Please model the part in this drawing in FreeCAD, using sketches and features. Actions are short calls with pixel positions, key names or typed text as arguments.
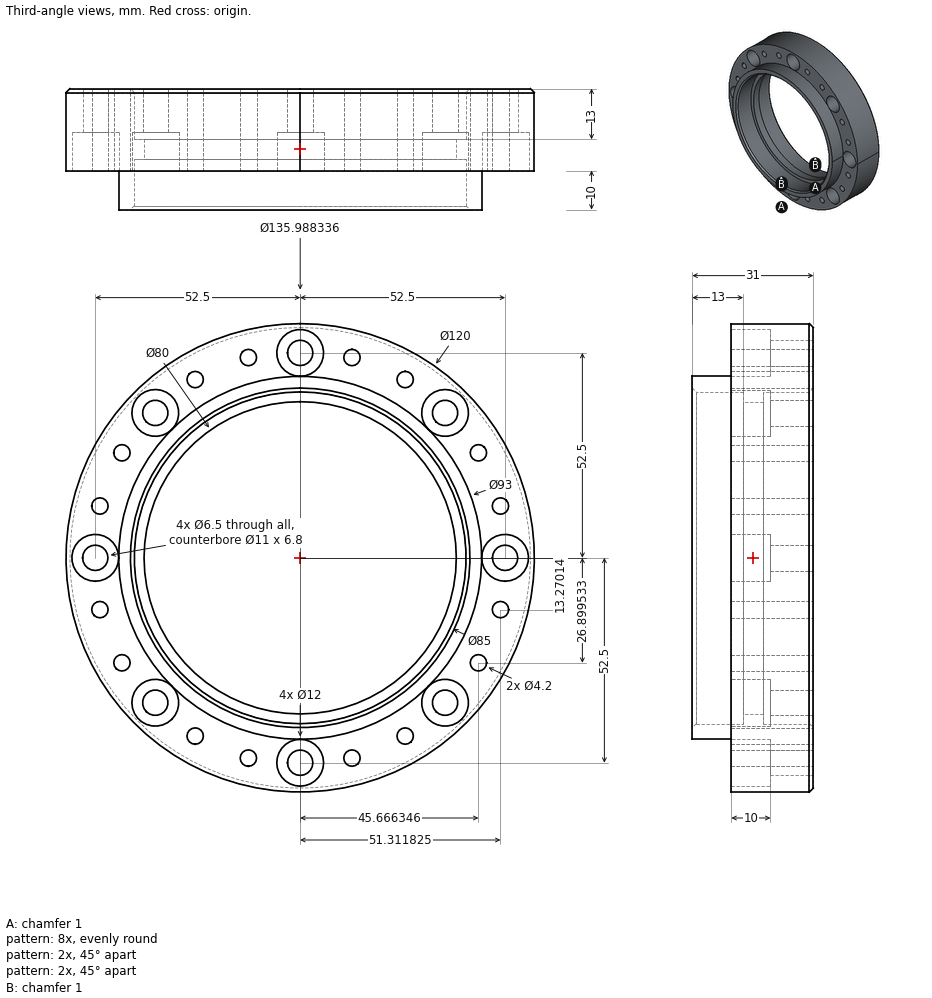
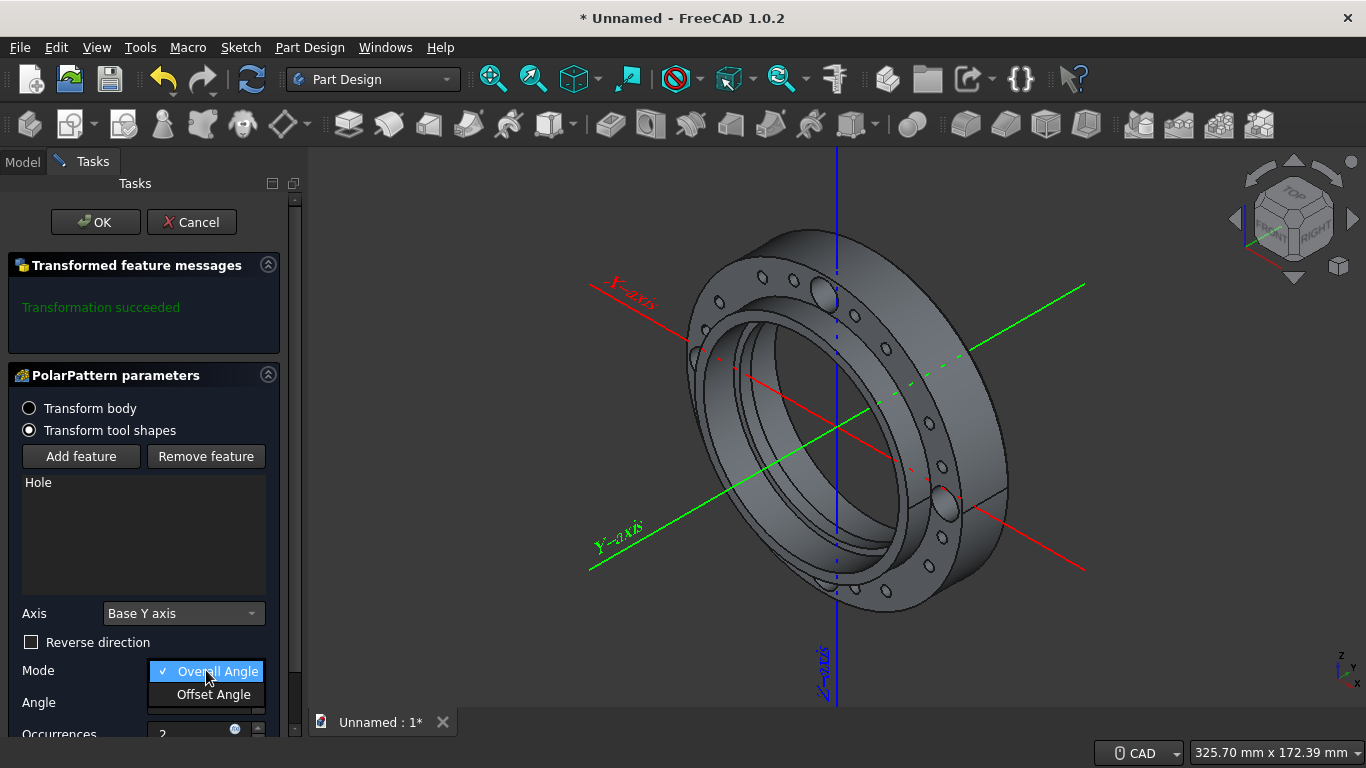
click(206, 694)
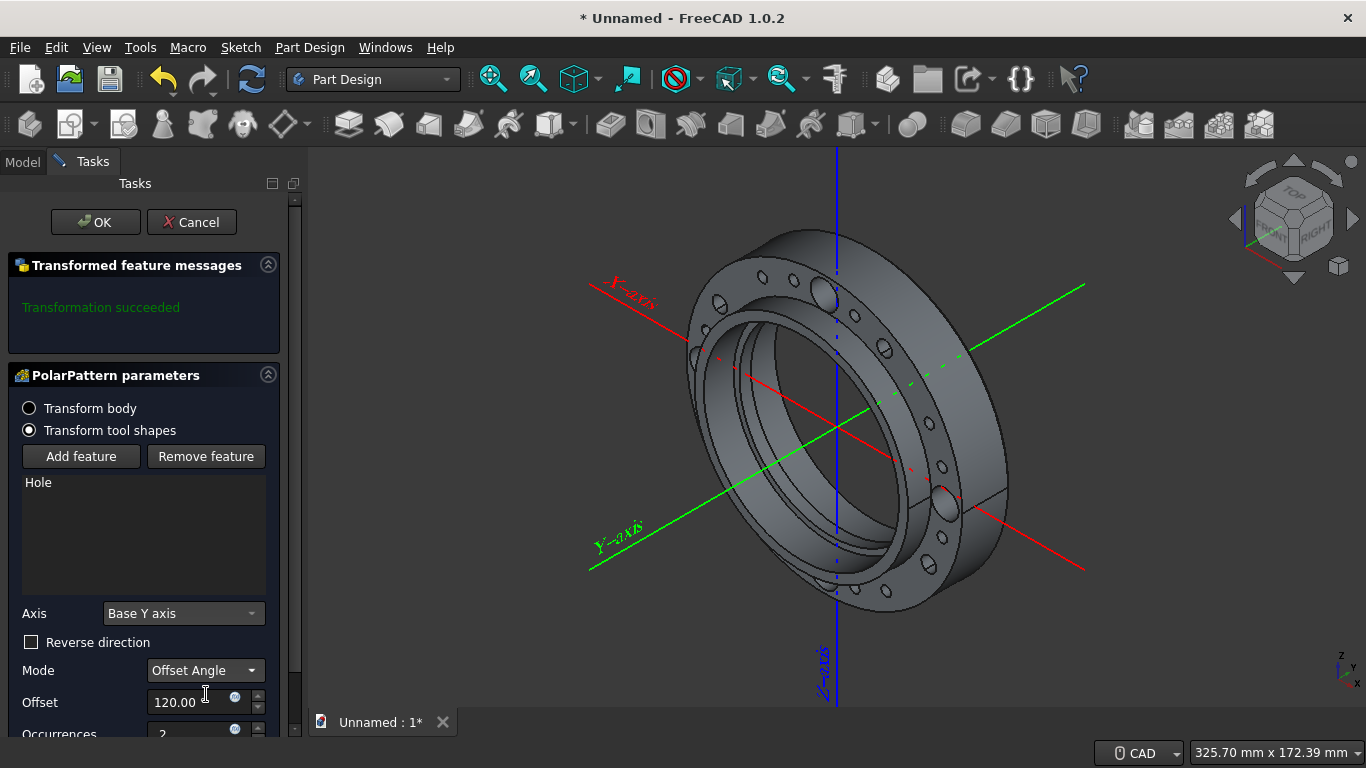
triple_click(198, 702)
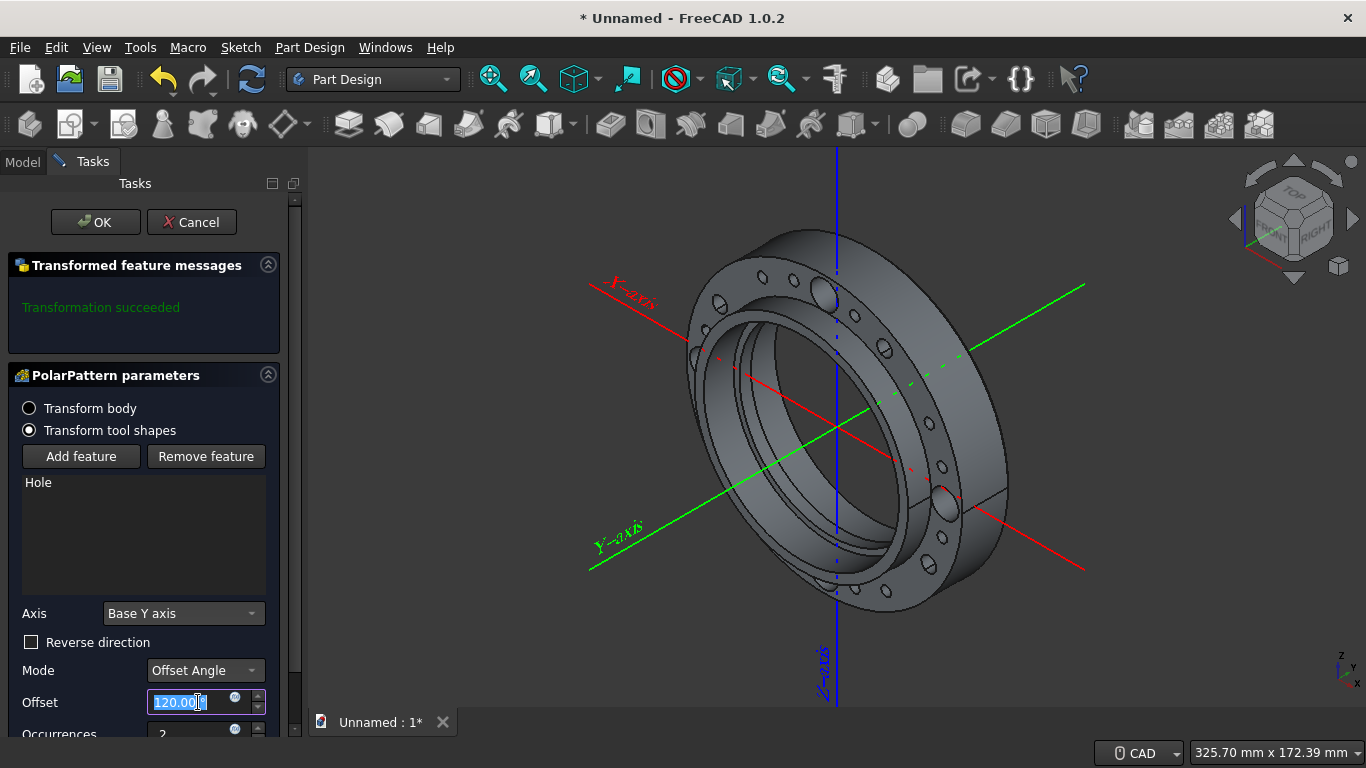
text(45)
key(Tab)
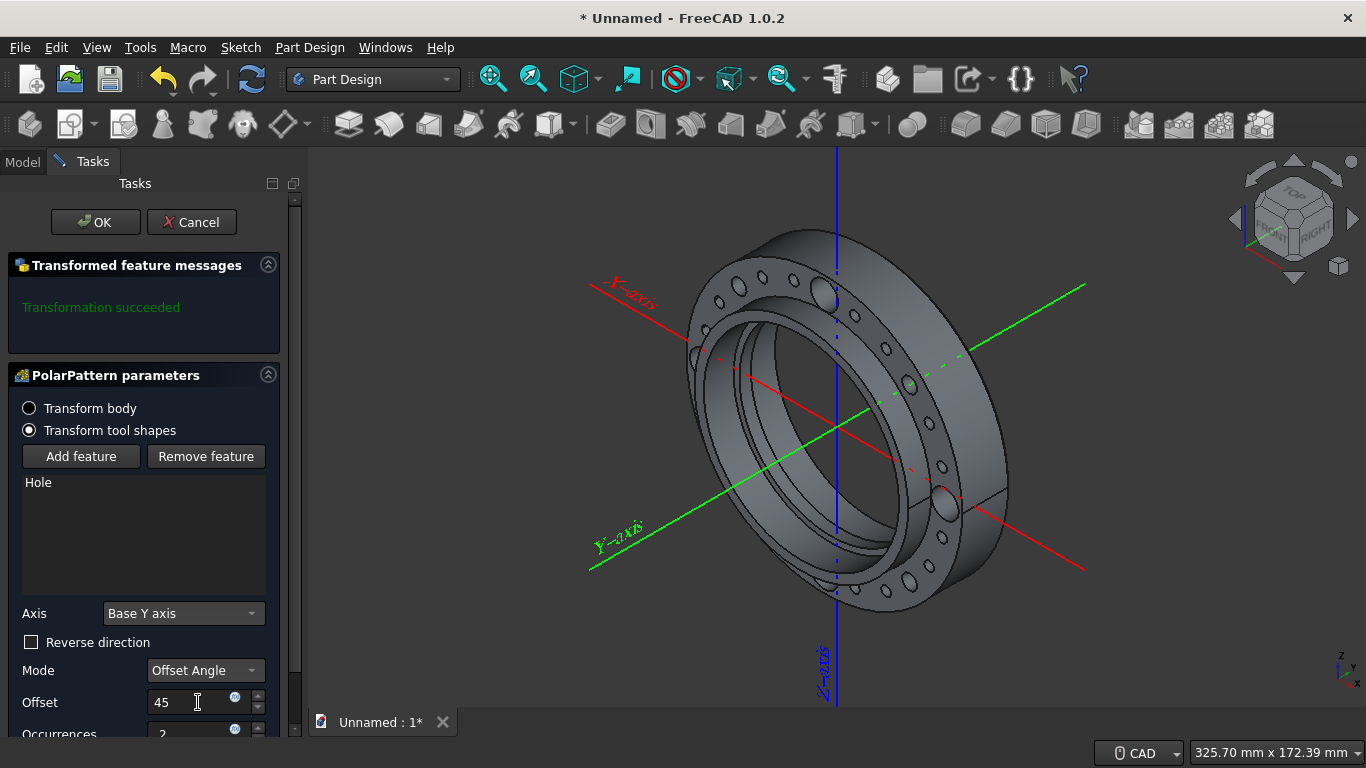
scroll(295, 464, down, 2)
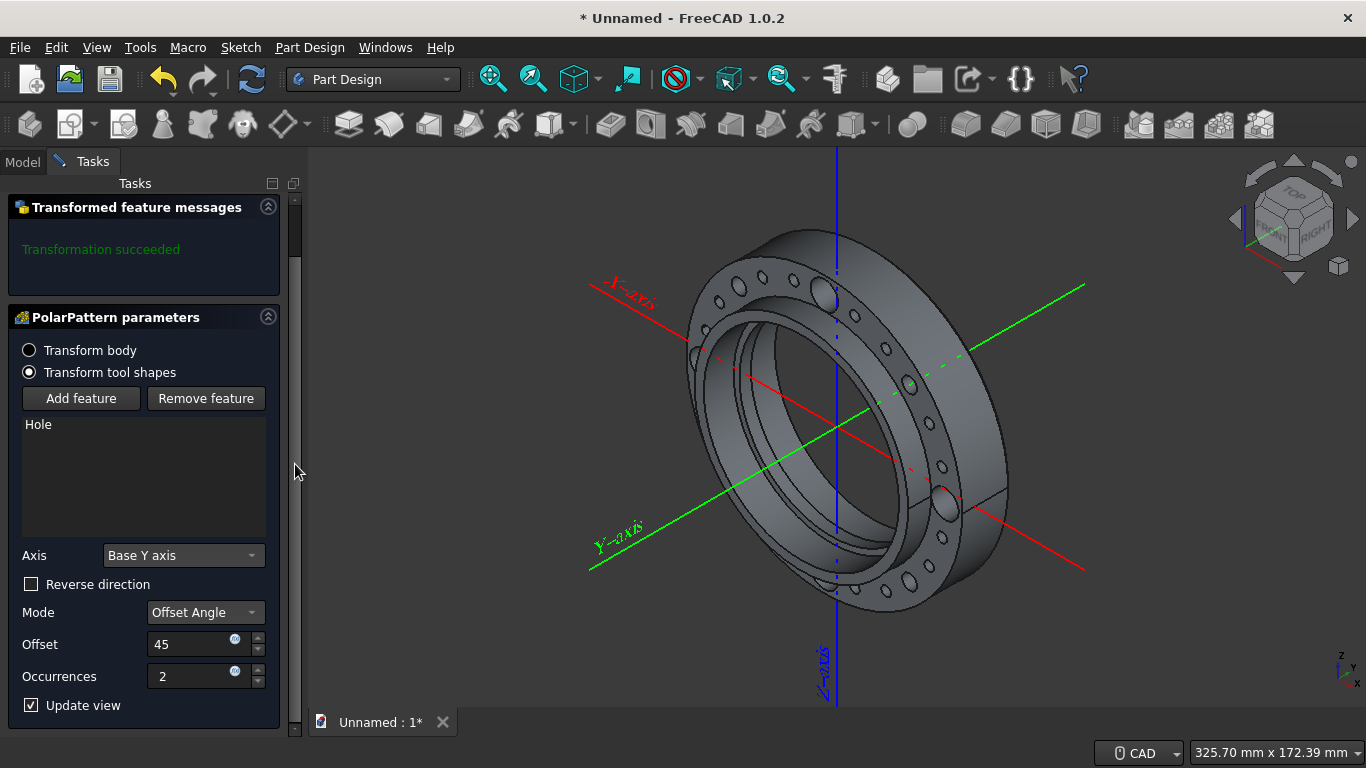
triple_click(198, 676)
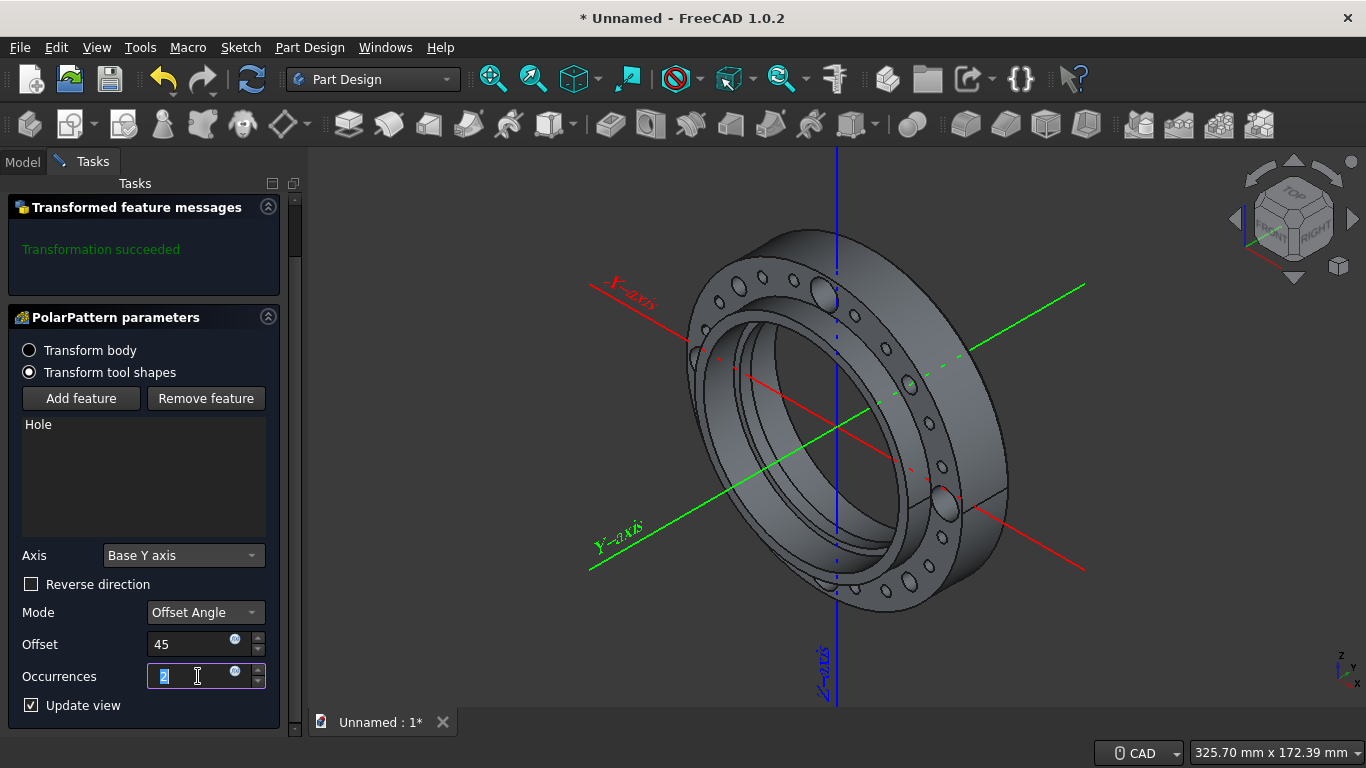
text(2)
key(Tab)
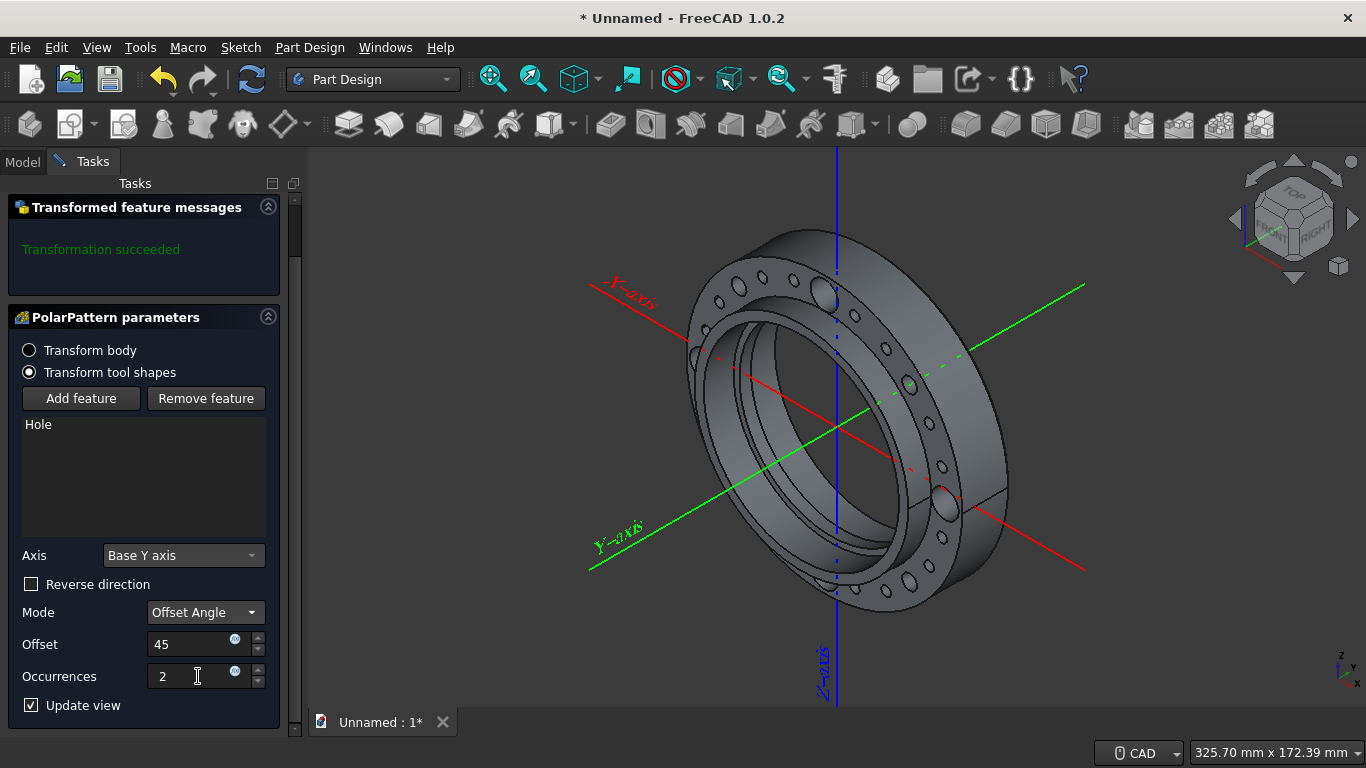
scroll(295, 464, up, 2)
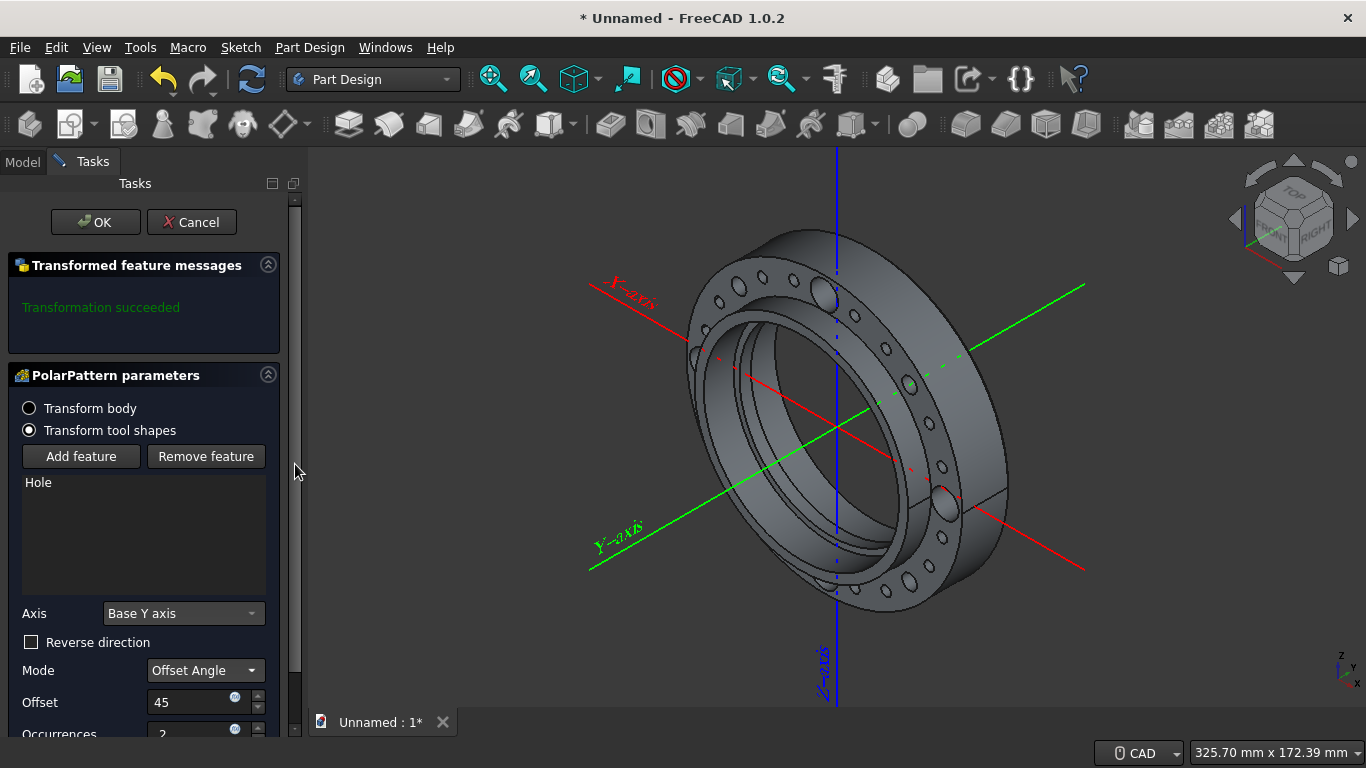
click(96, 222)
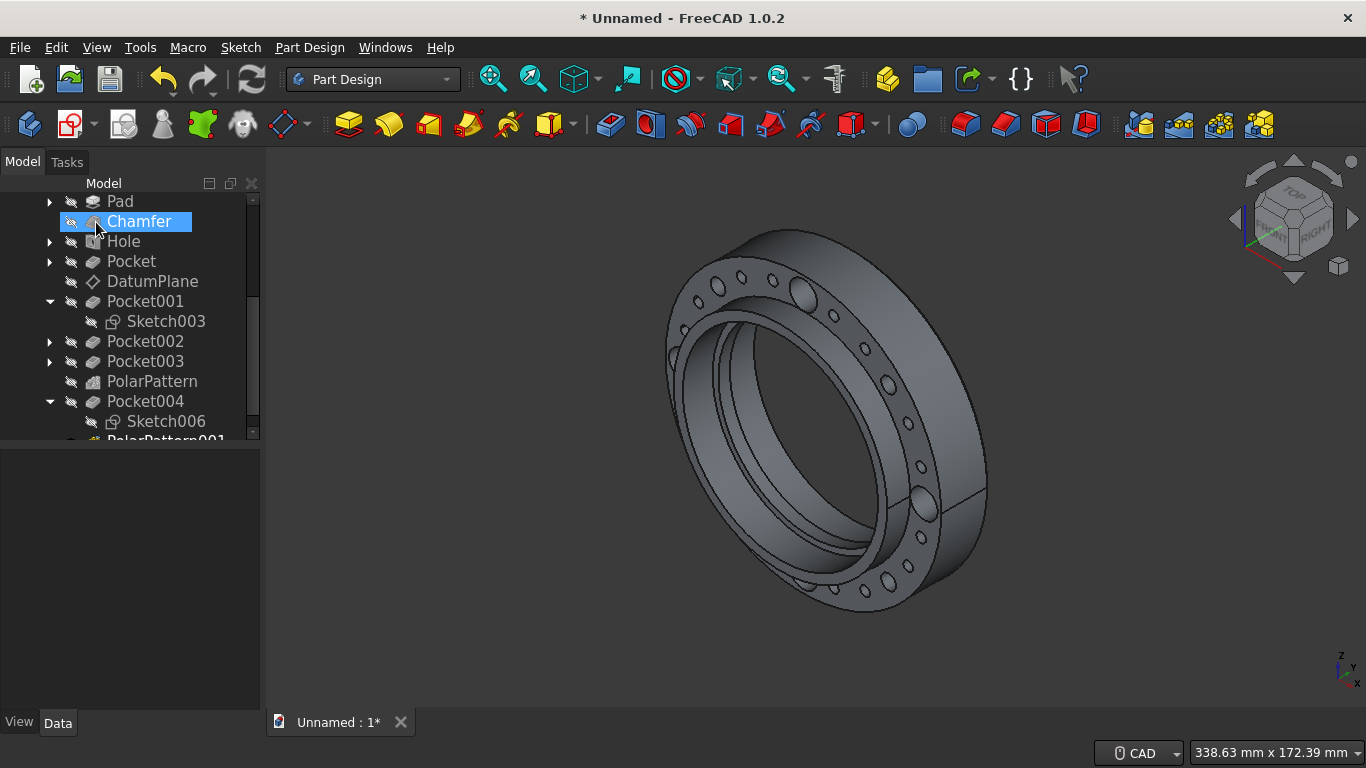
click(116, 402)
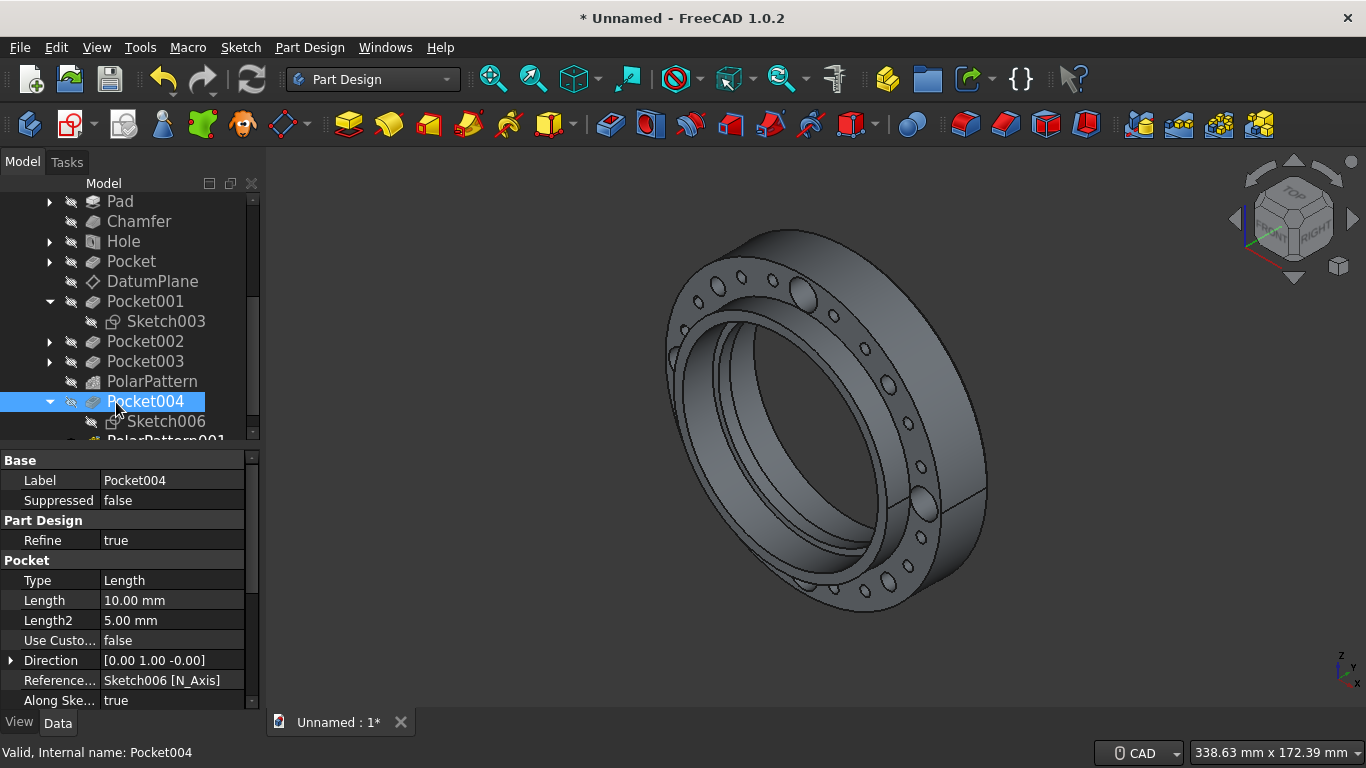
click(1220, 124)